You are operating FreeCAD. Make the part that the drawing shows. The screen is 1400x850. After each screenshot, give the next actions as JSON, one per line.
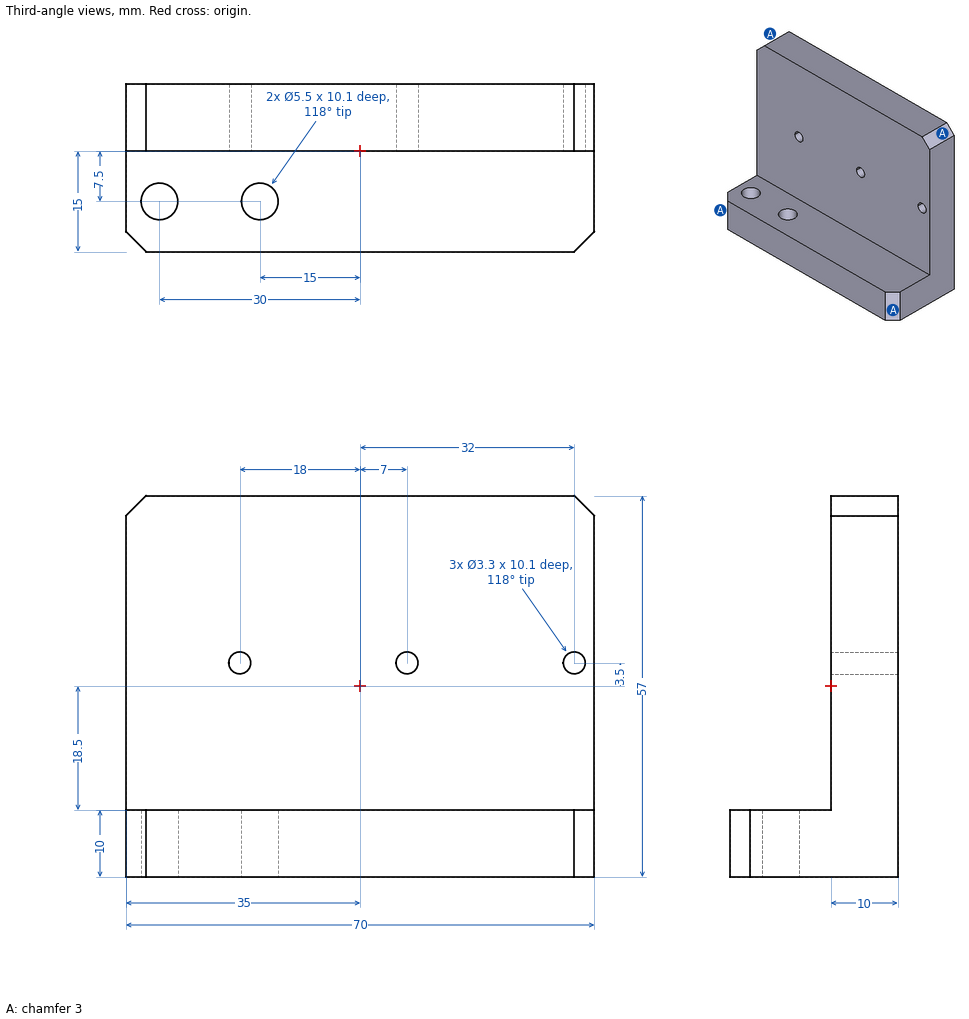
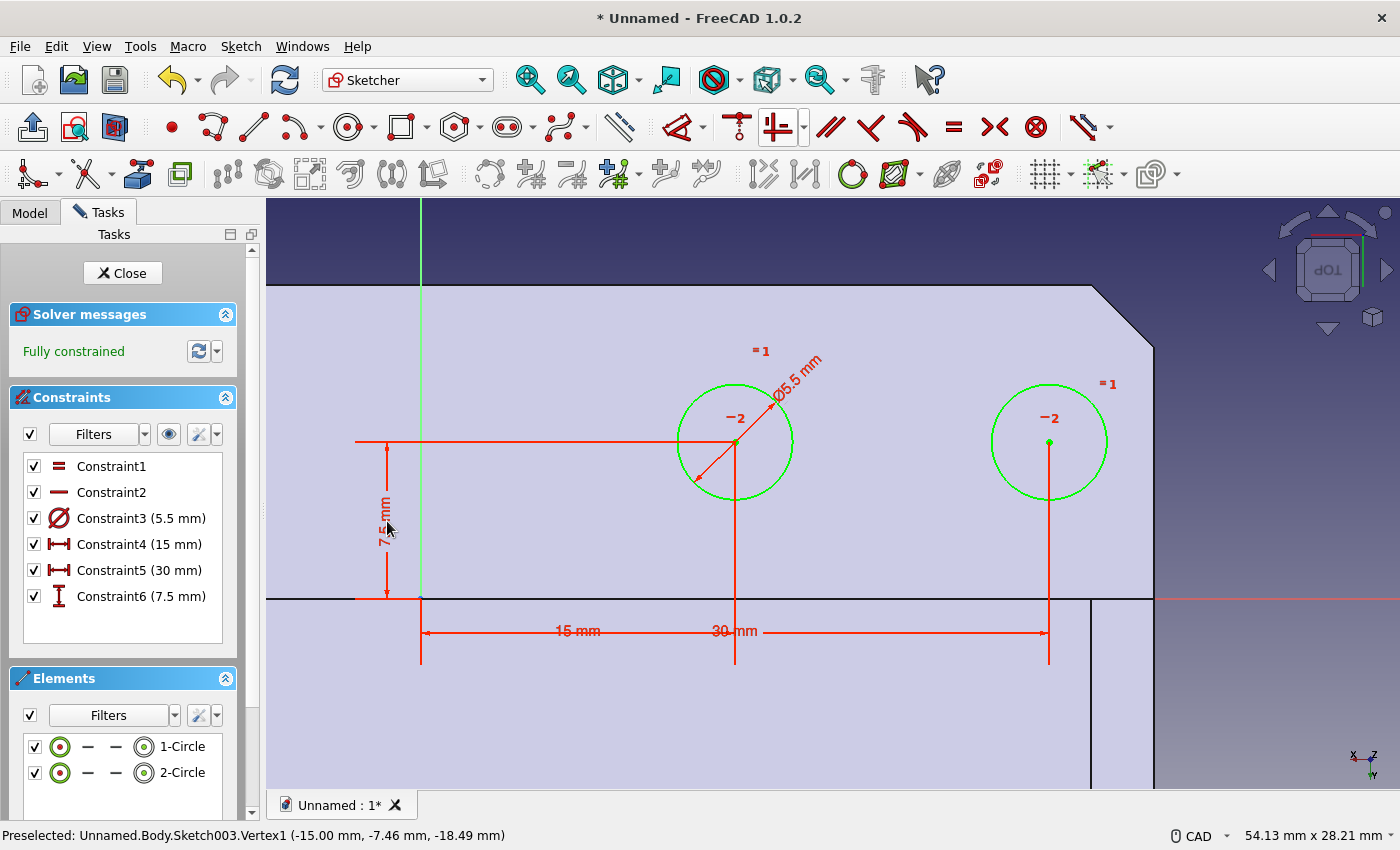
{"action": "left_click", "coordinate": [123, 273]}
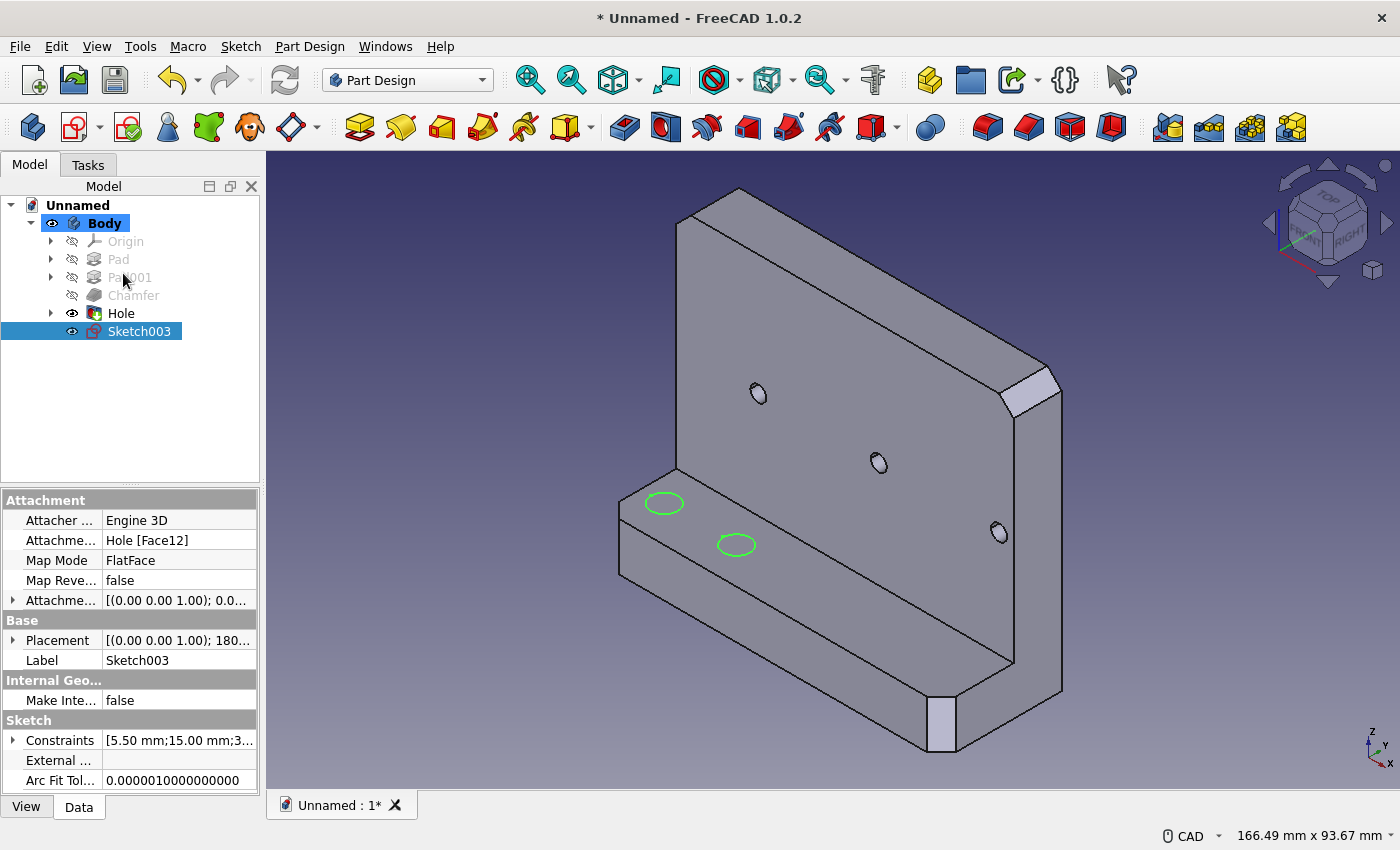
{"action": "left_click", "coordinate": [666, 128]}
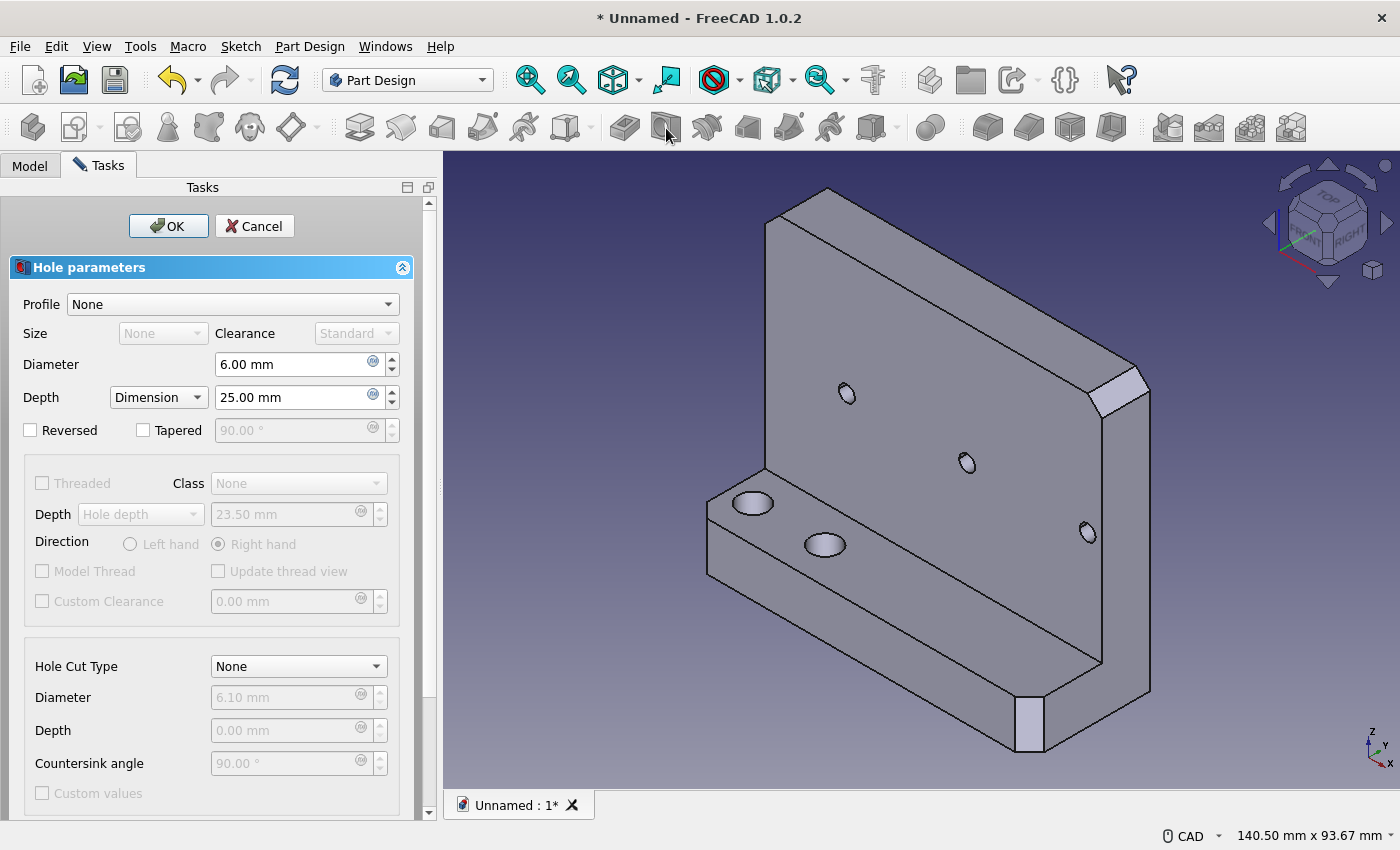
{"action": "triple_click", "coordinate": [300, 364]}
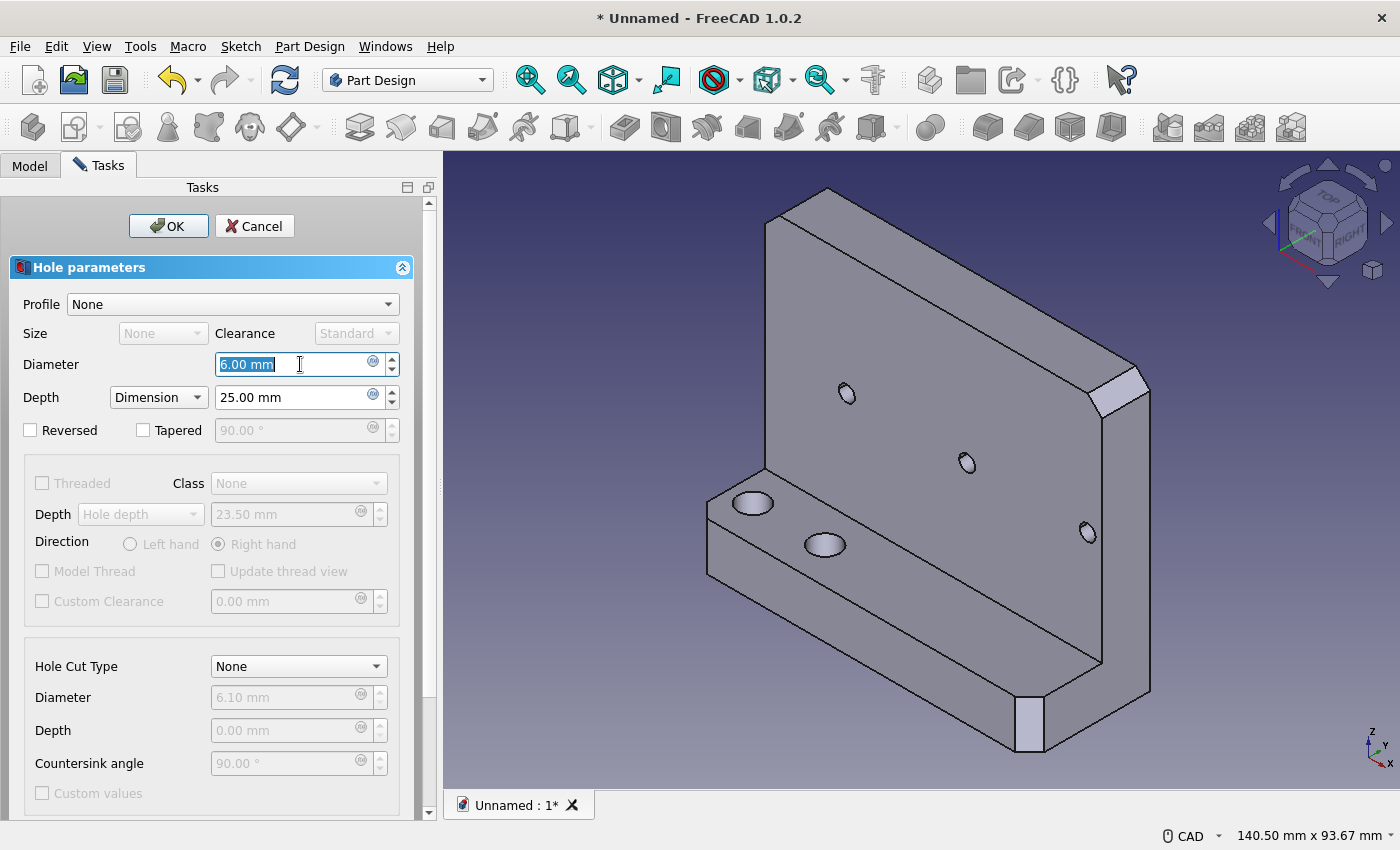
{"action": "type", "text": "5.5"}
{"action": "key", "text": "Tab"}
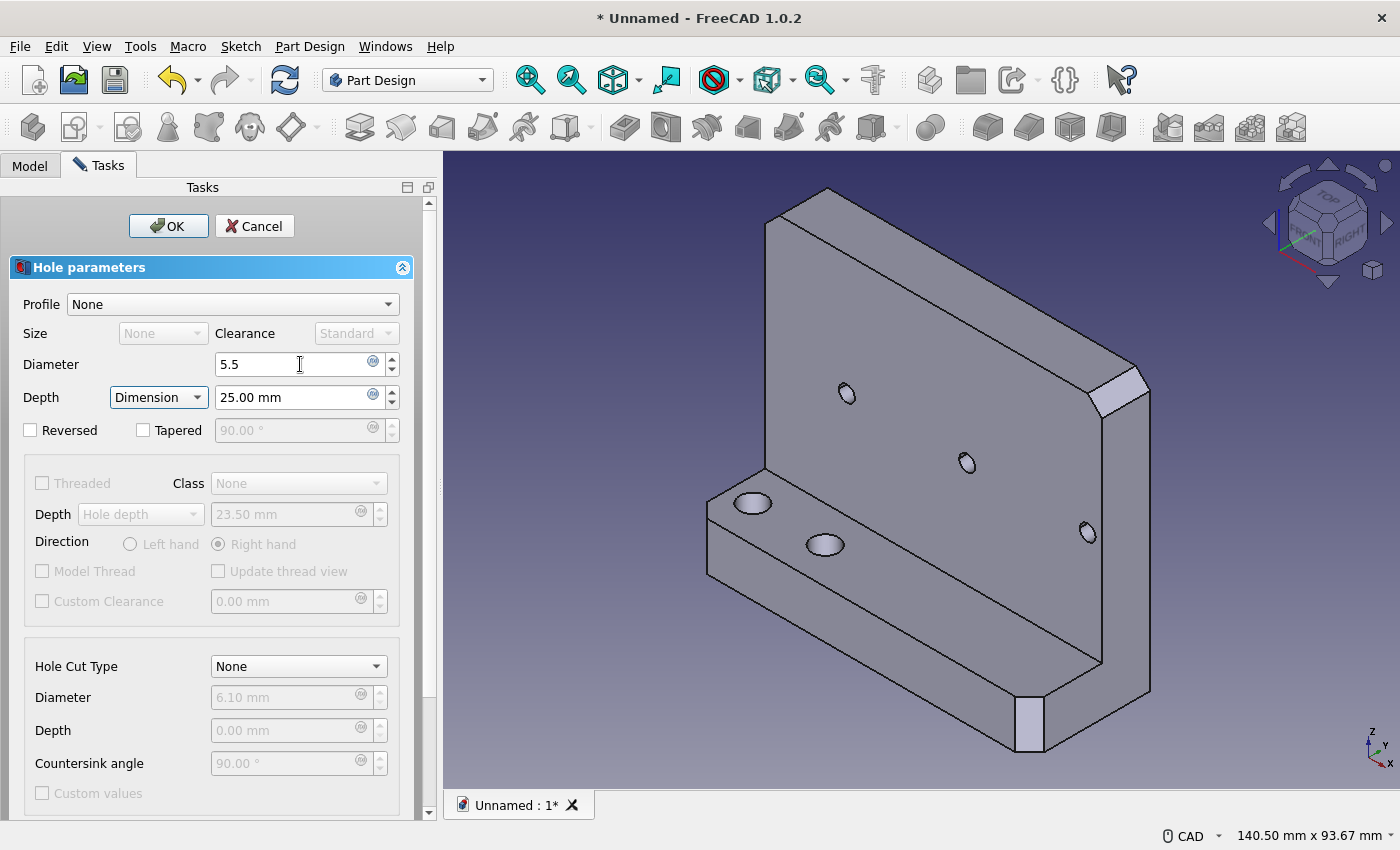
{"action": "triple_click", "coordinate": [300, 398]}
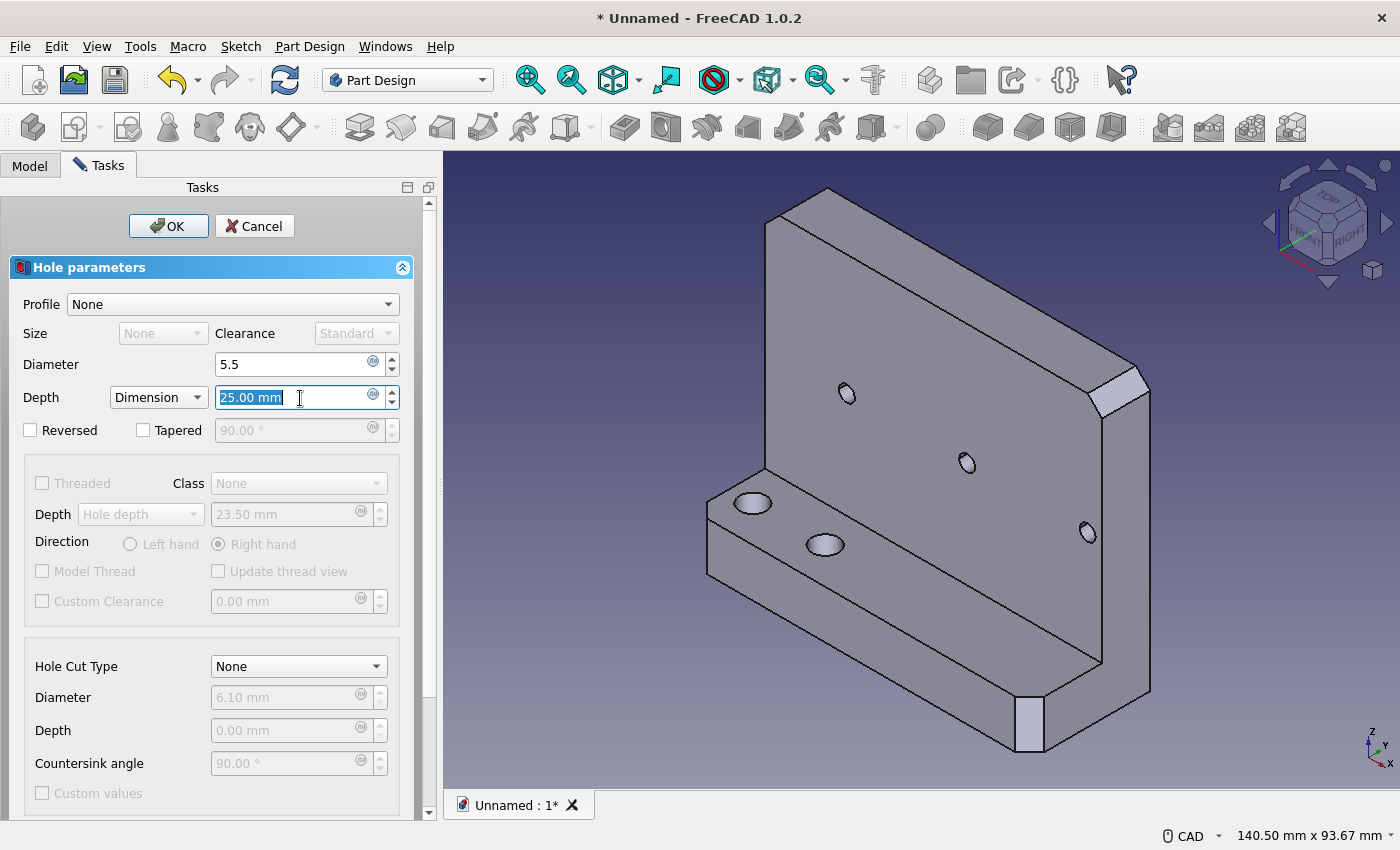
{"action": "type", "text": "10.1"}
{"action": "key", "text": "Tab"}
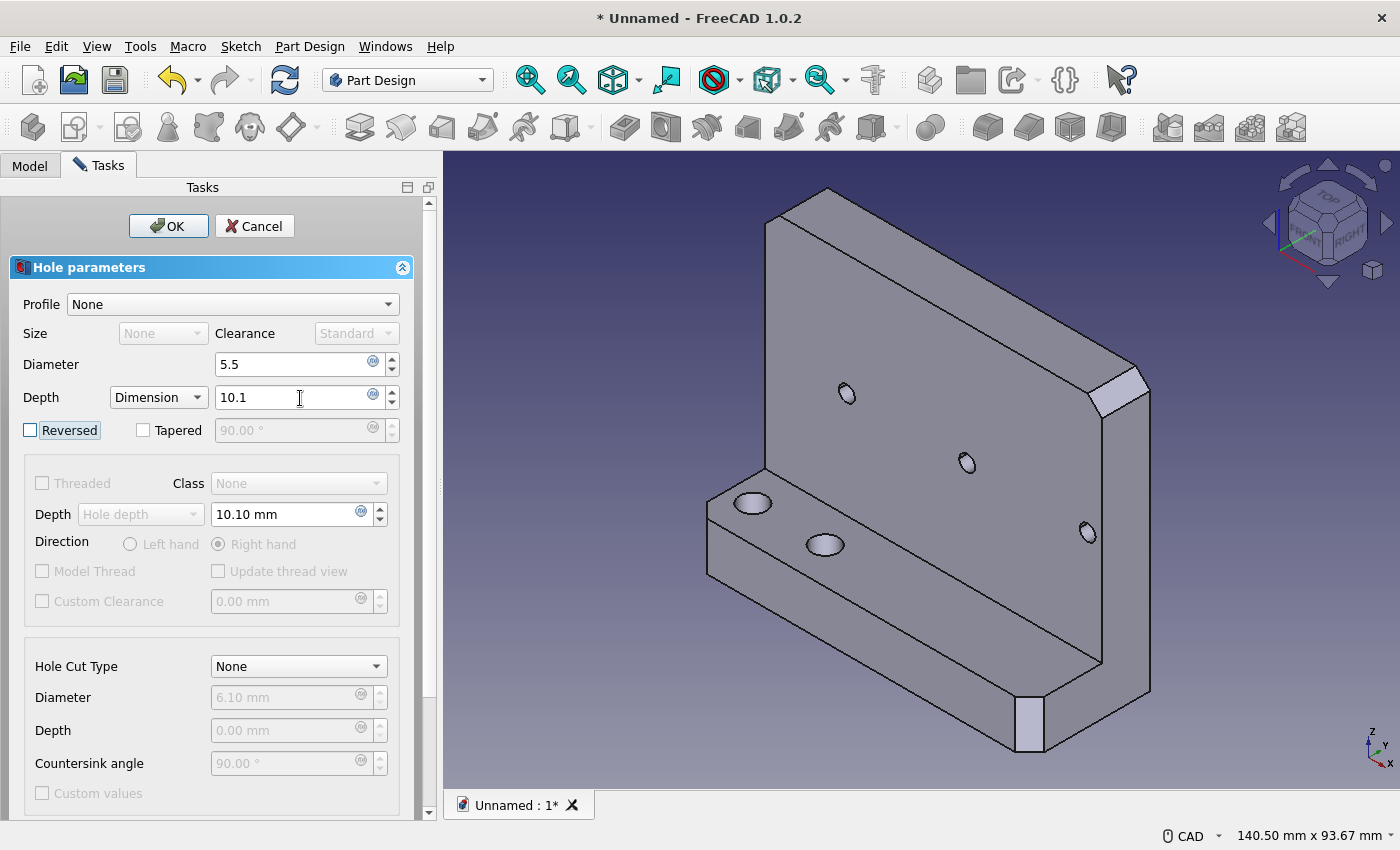
{"action": "left_click", "coordinate": [169, 226]}